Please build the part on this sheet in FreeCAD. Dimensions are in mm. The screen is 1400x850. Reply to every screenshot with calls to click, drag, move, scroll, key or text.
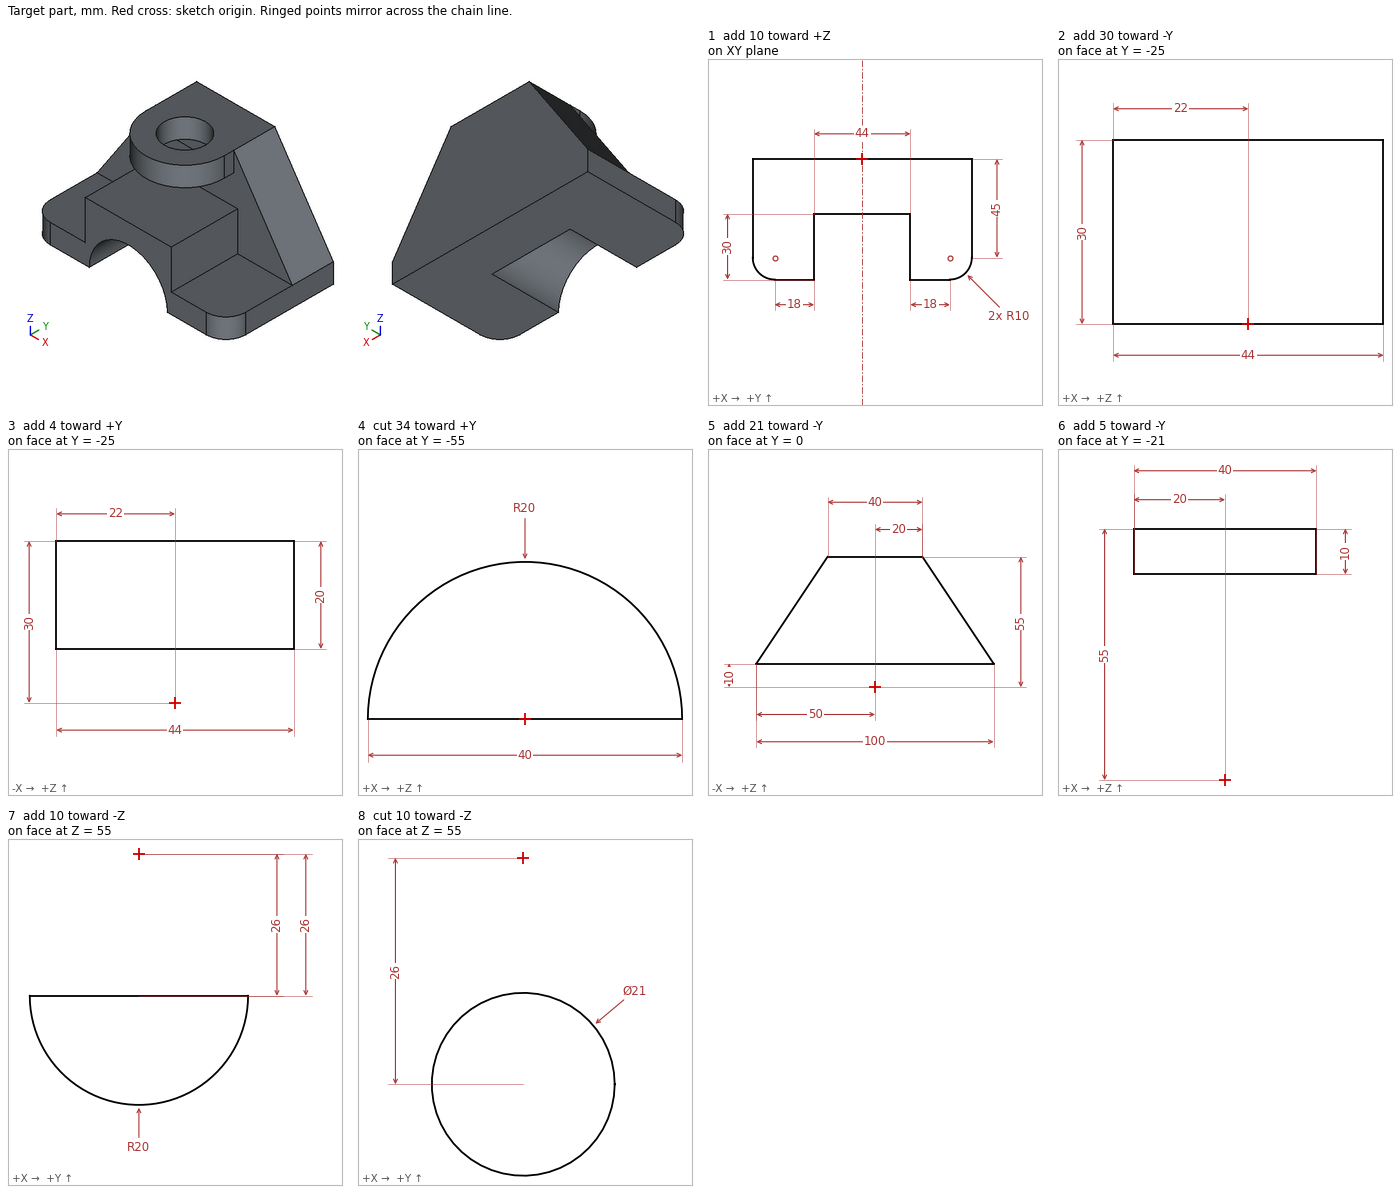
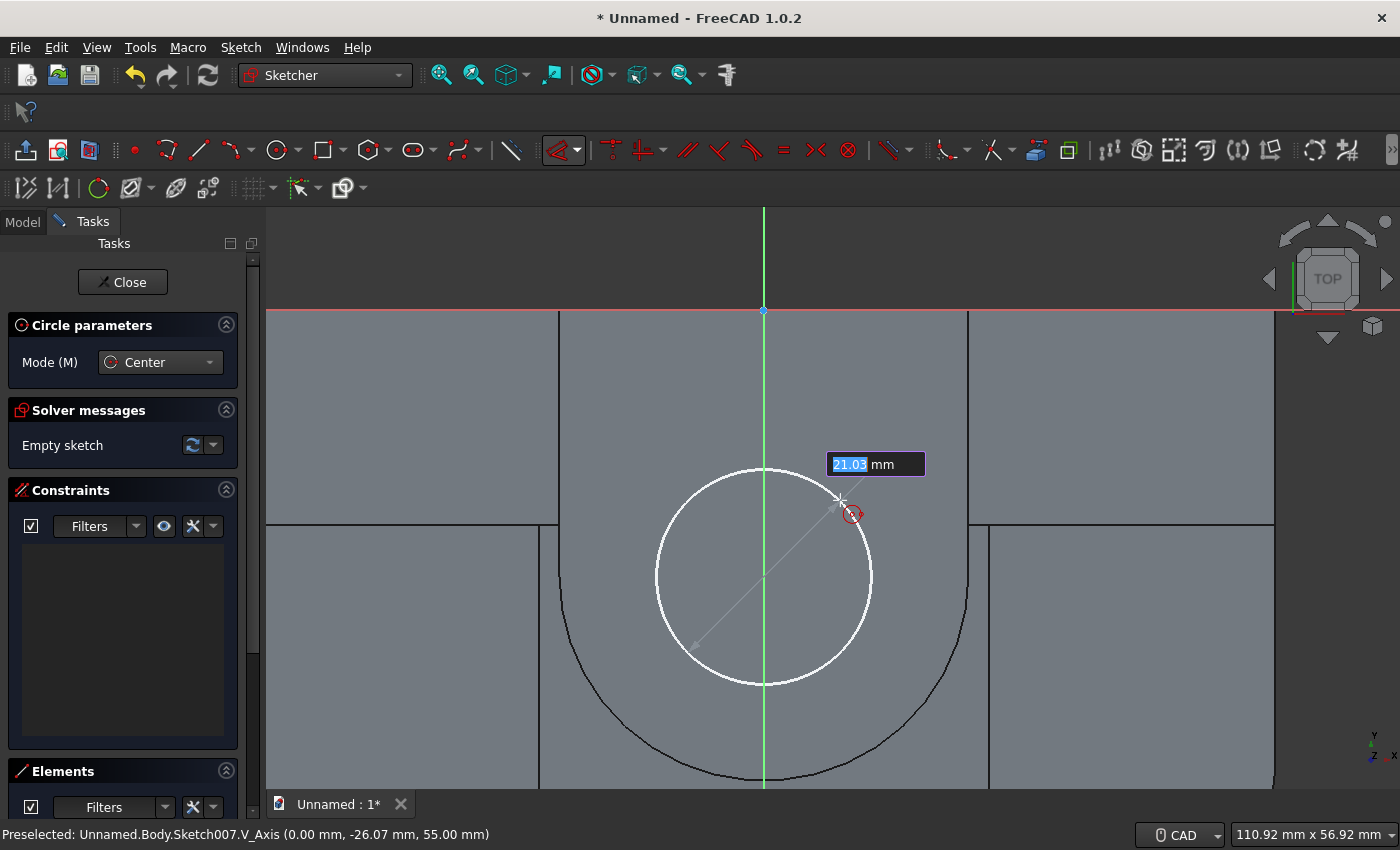
text(21)
key(Return)
key(Escape)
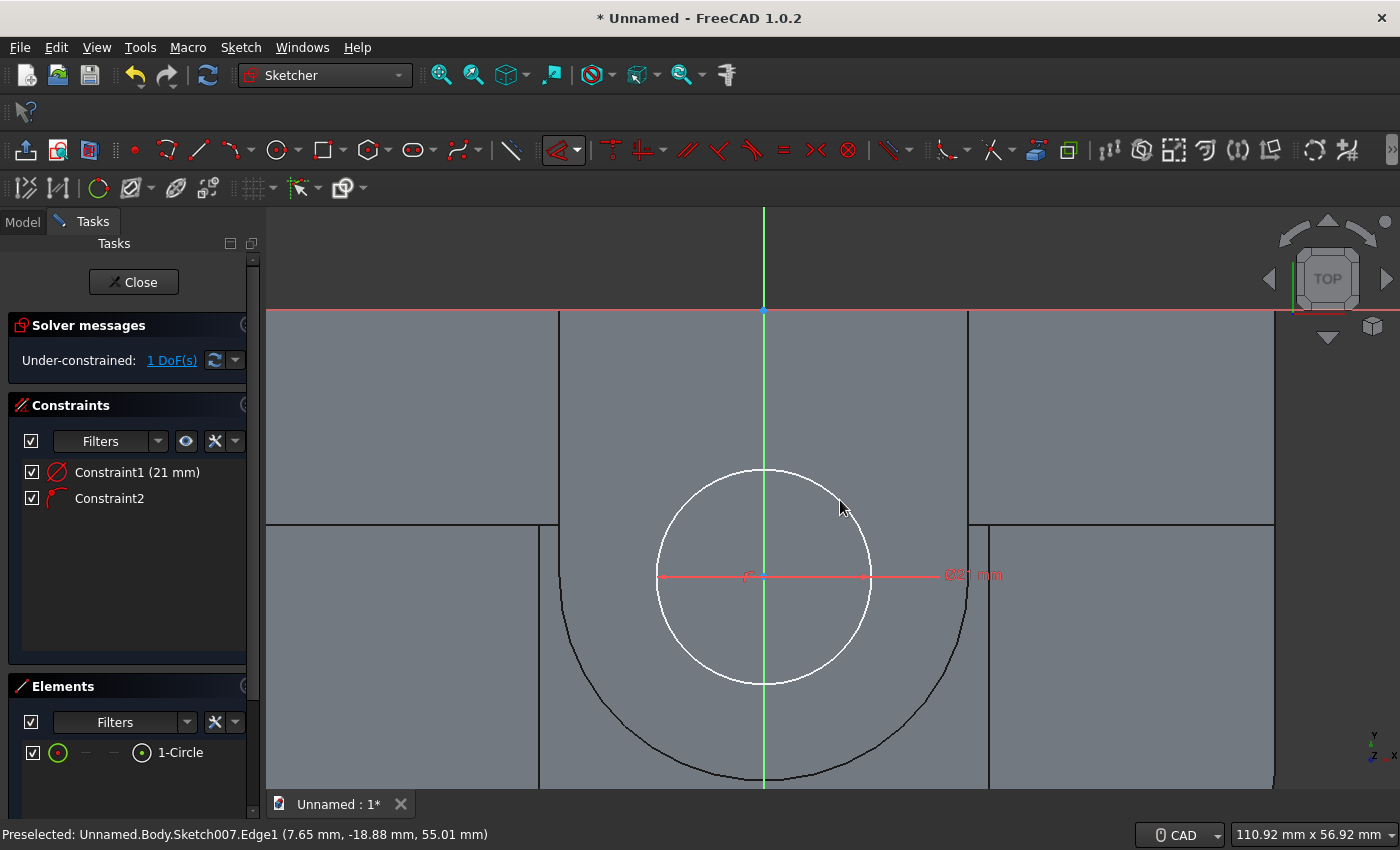
click(764, 577)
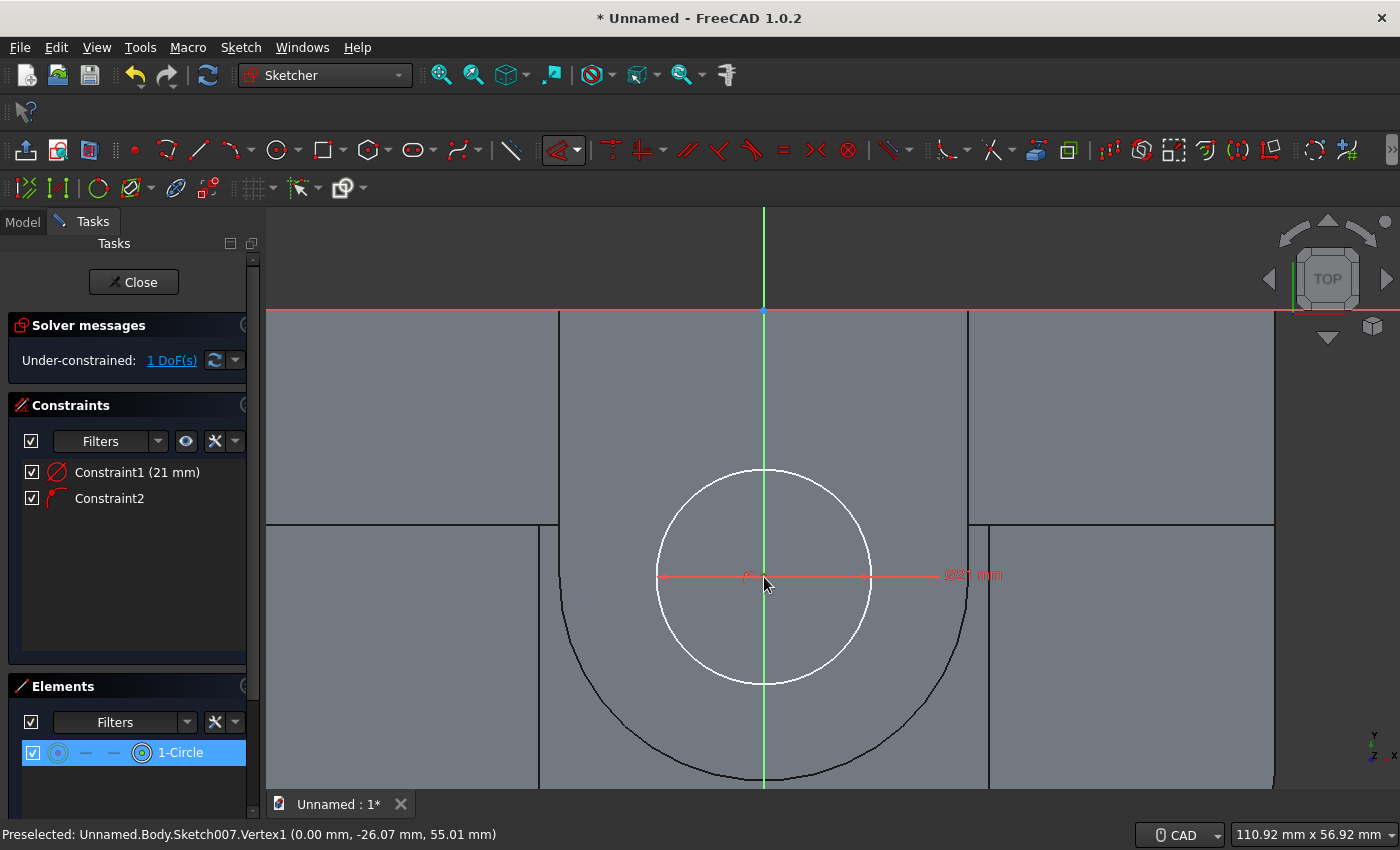
key(i)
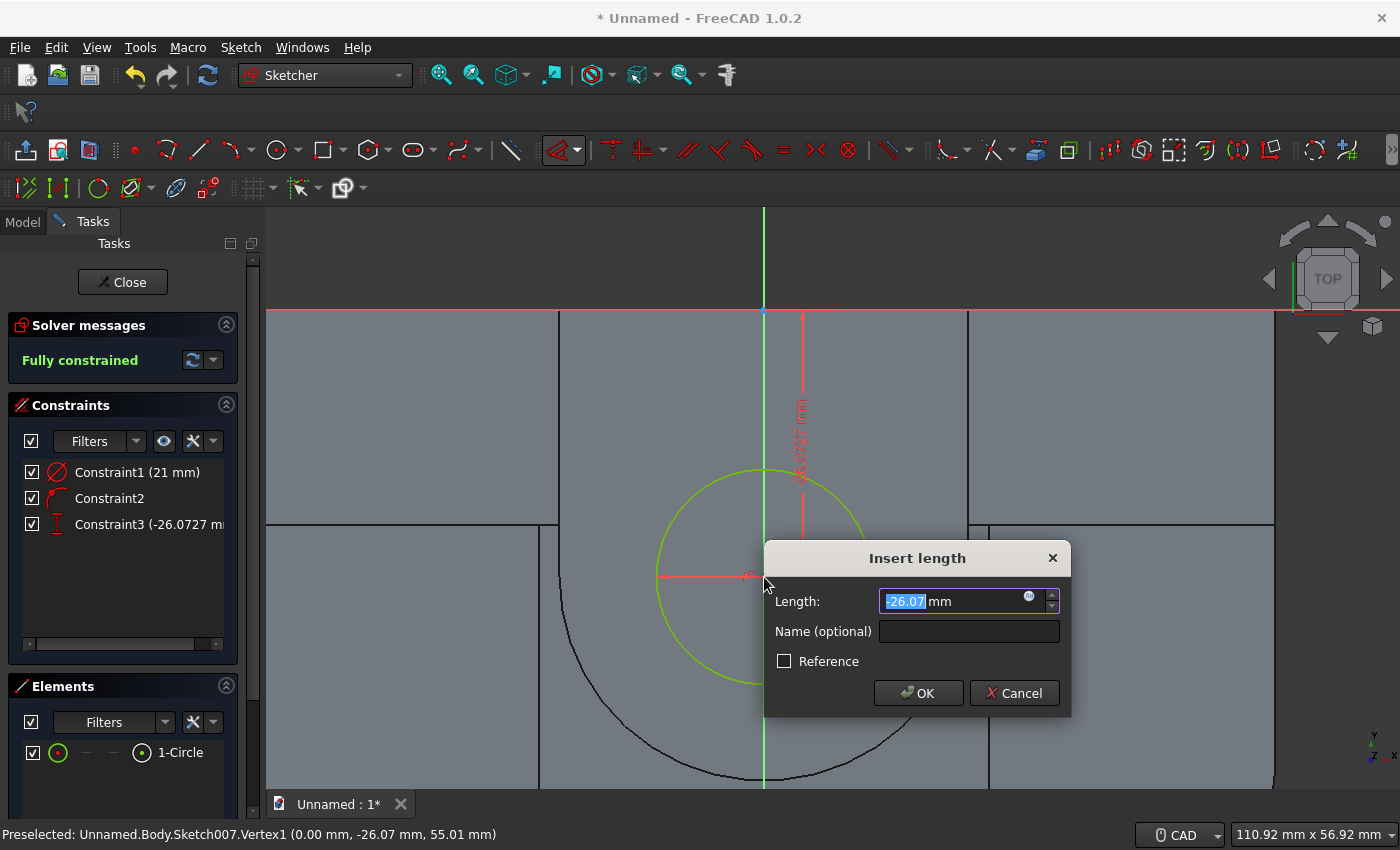
text(-26)
key(Return)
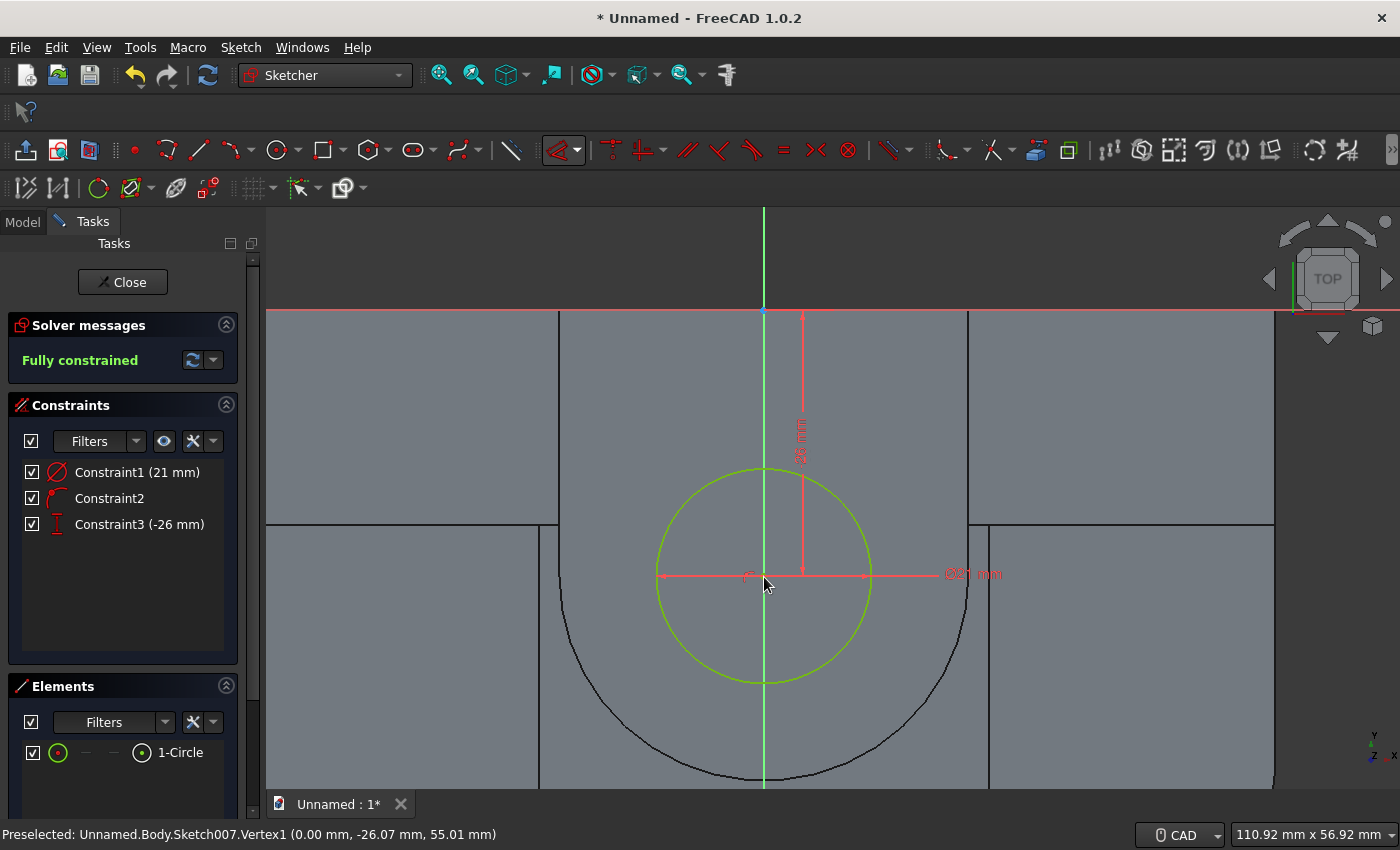
click(123, 282)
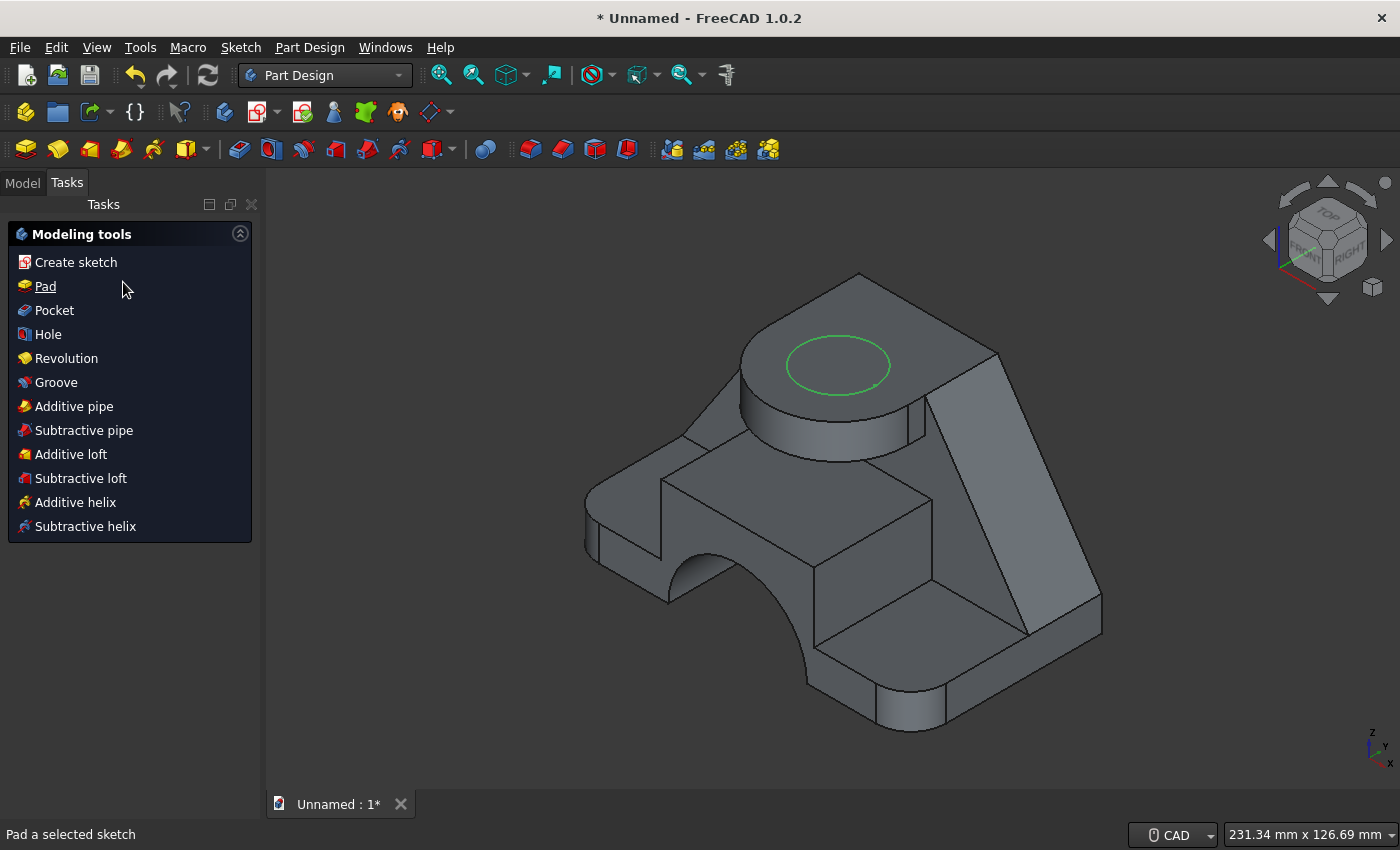
click(240, 150)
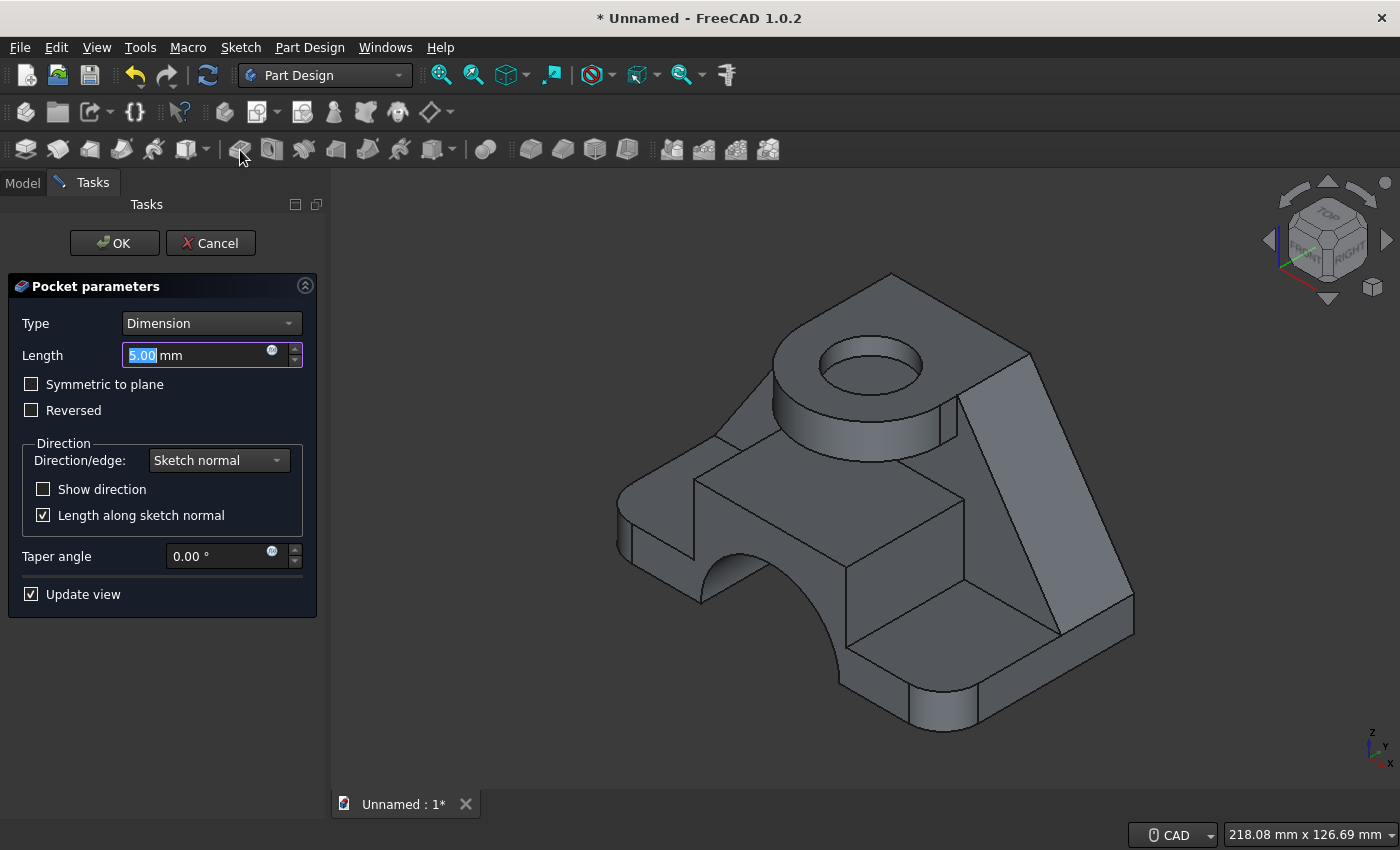
text(10)
key(Tab)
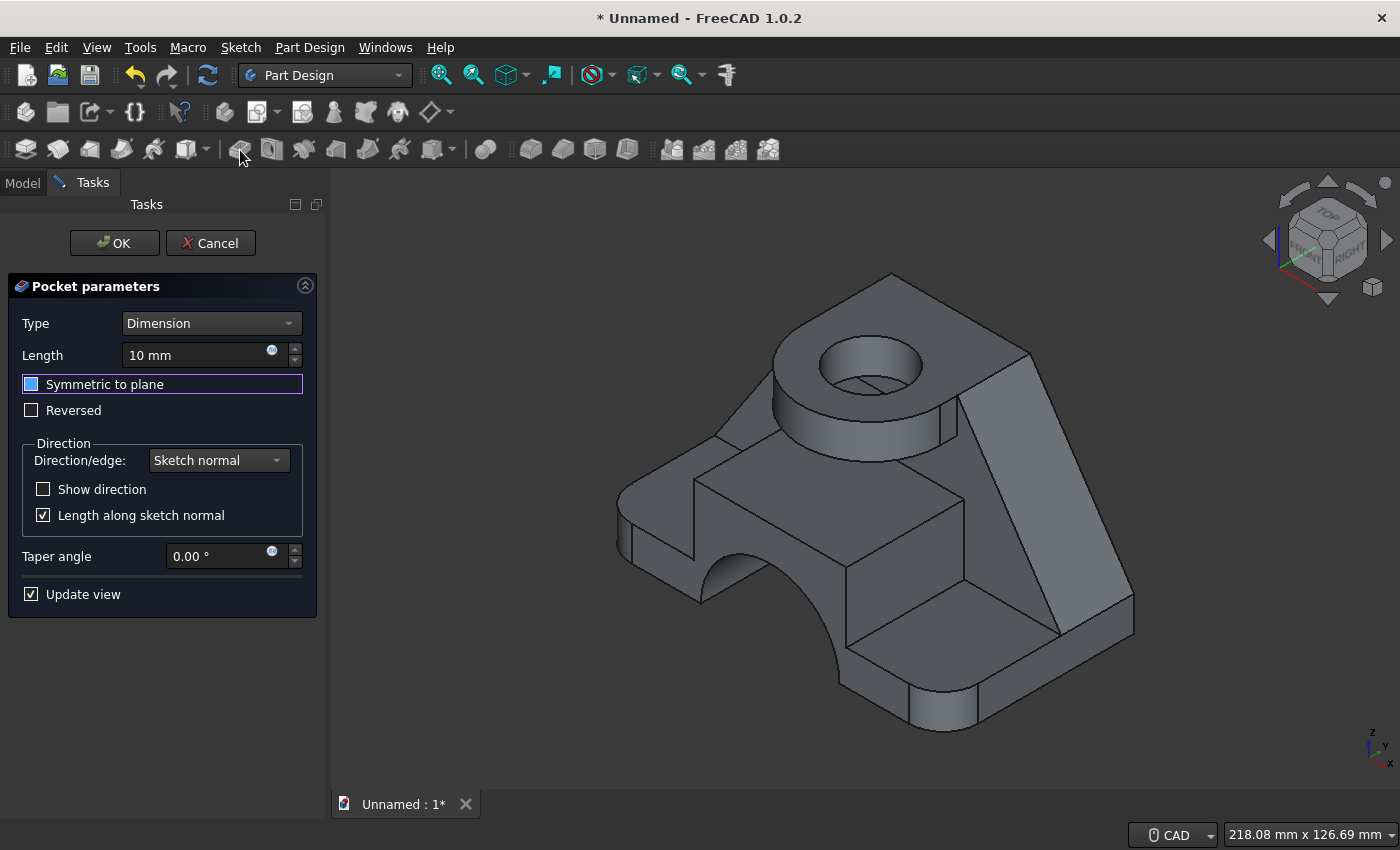
click(115, 243)